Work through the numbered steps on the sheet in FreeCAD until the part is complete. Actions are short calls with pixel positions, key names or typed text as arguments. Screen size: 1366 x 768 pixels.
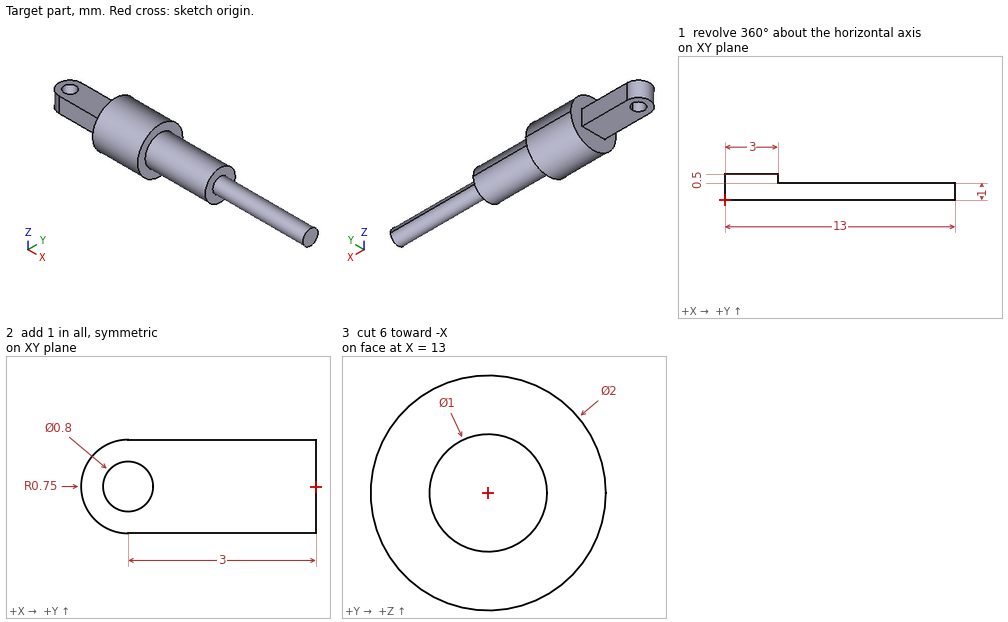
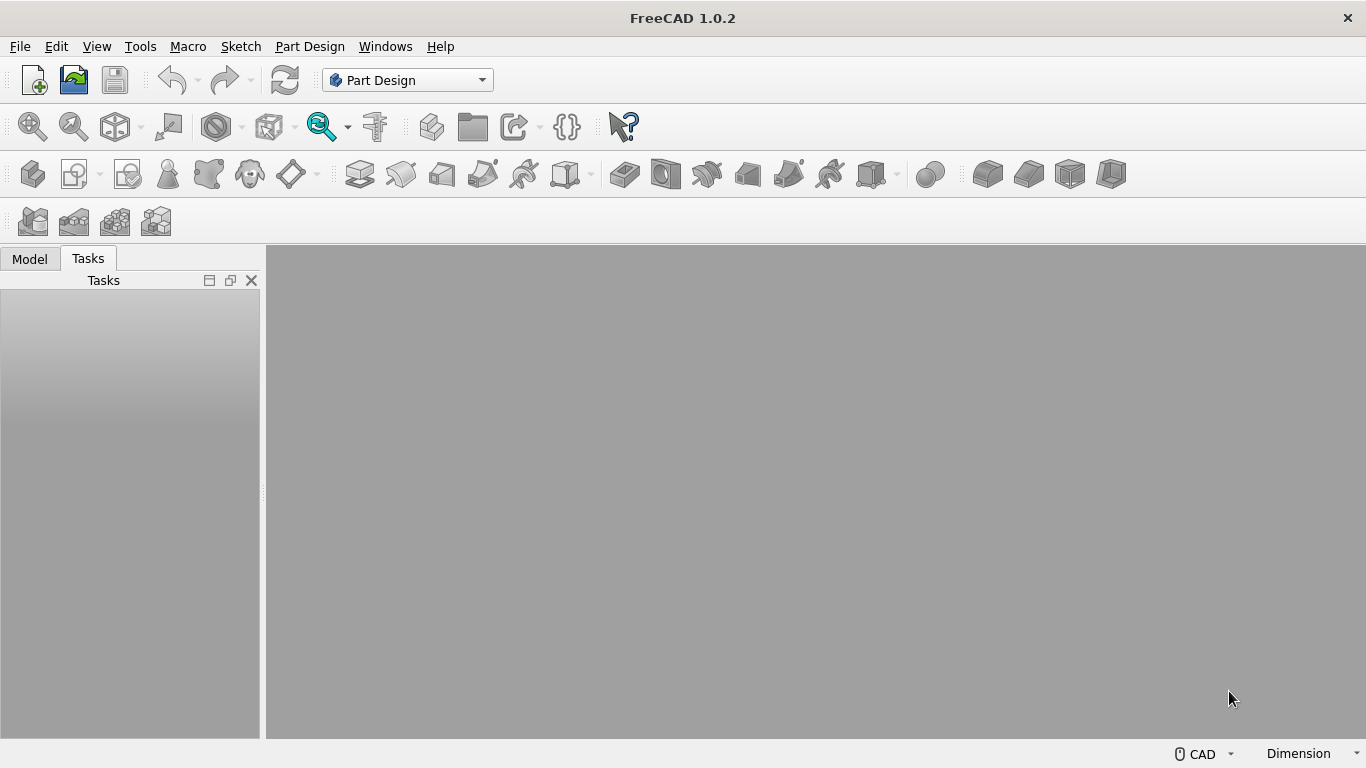
key(ctrl+n)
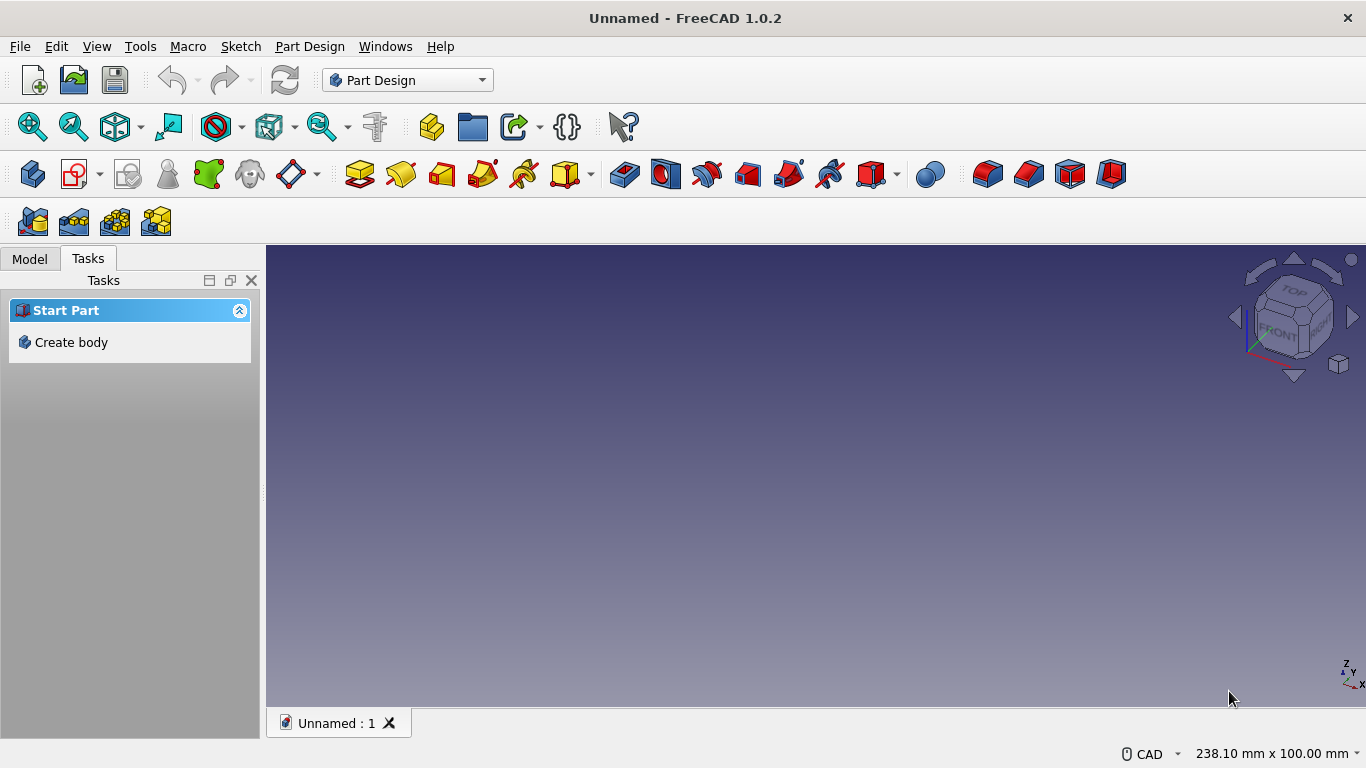
click(74, 174)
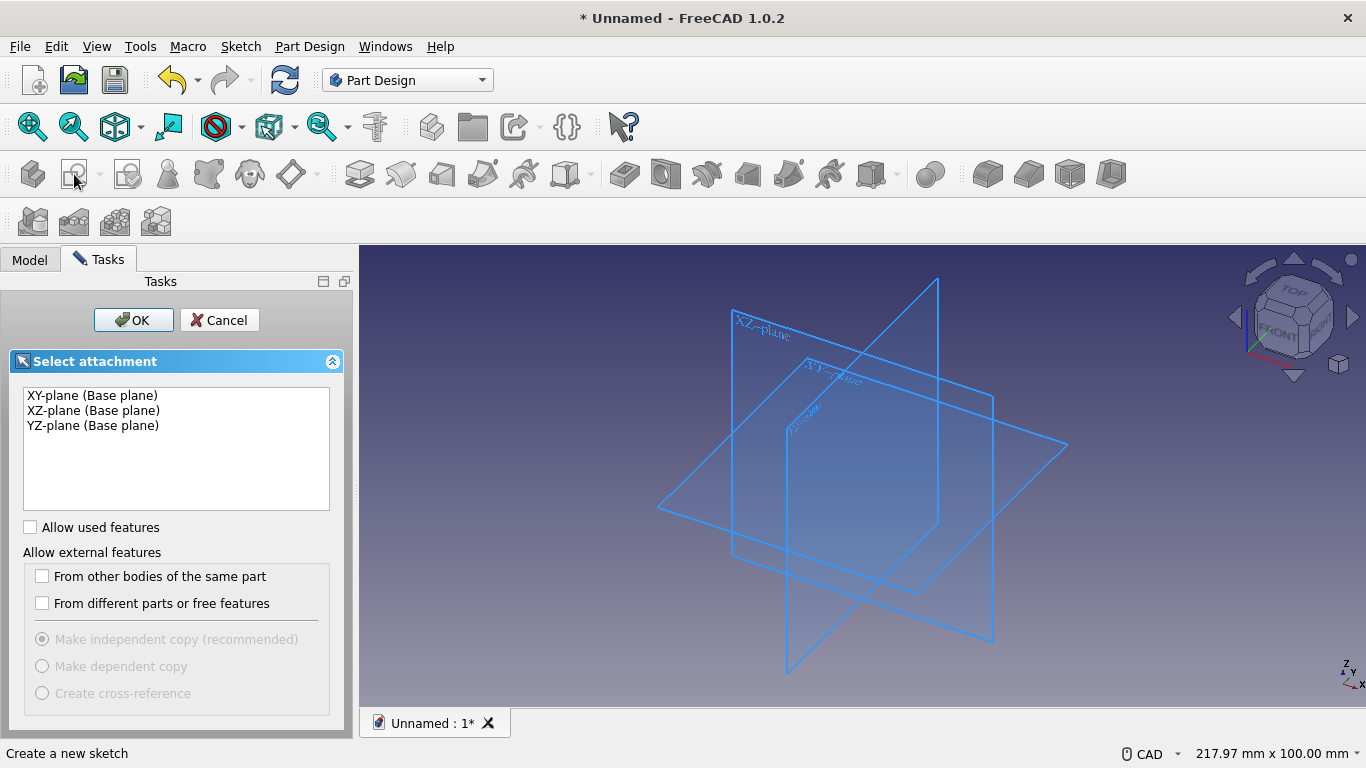
click(84, 396)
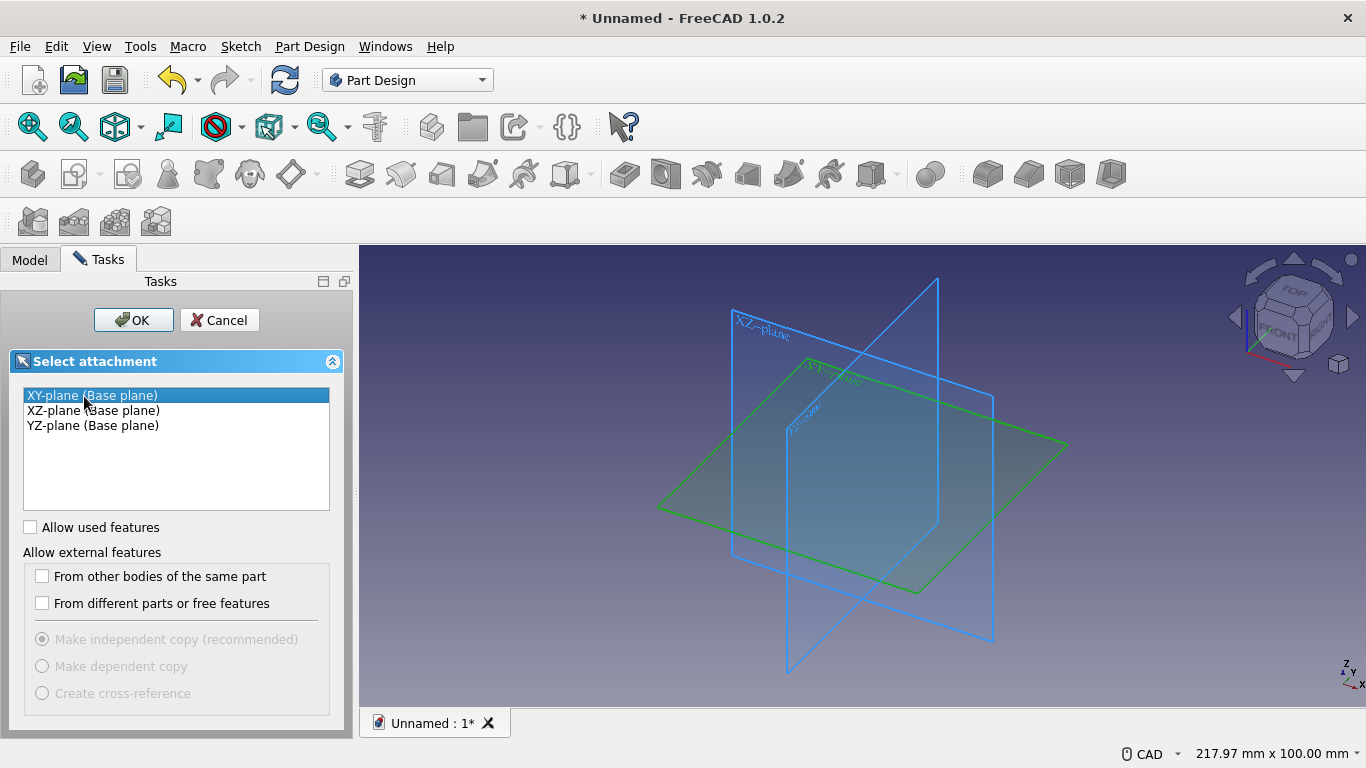
click(134, 320)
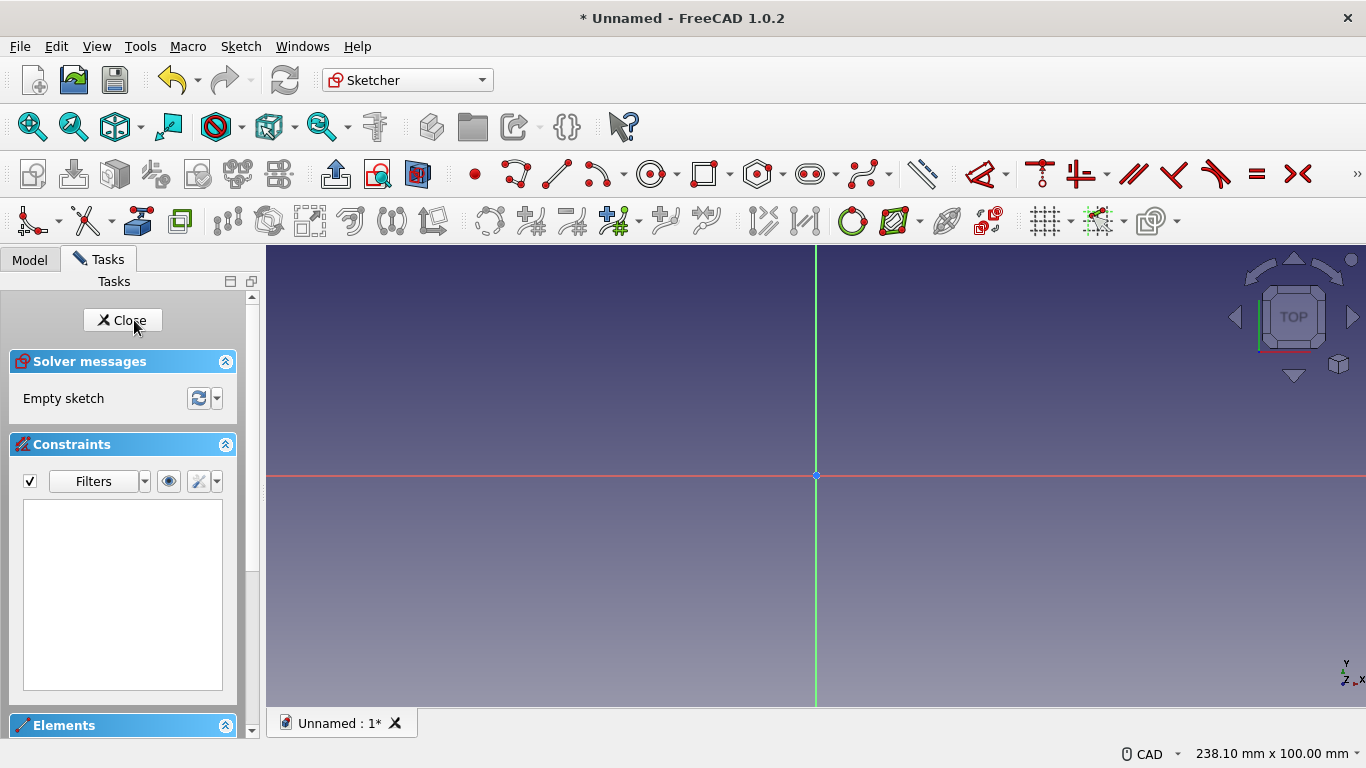
scroll(856, 472, up, 12)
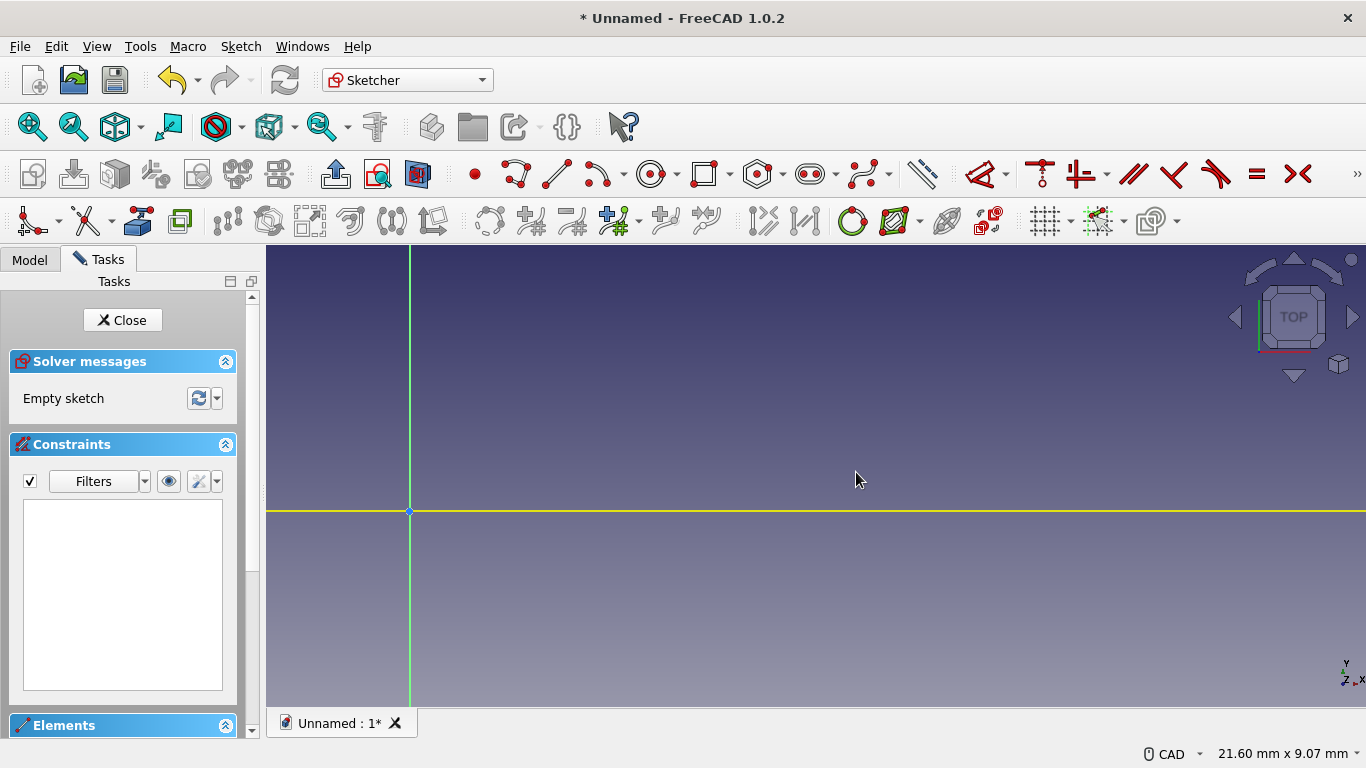
click(516, 174)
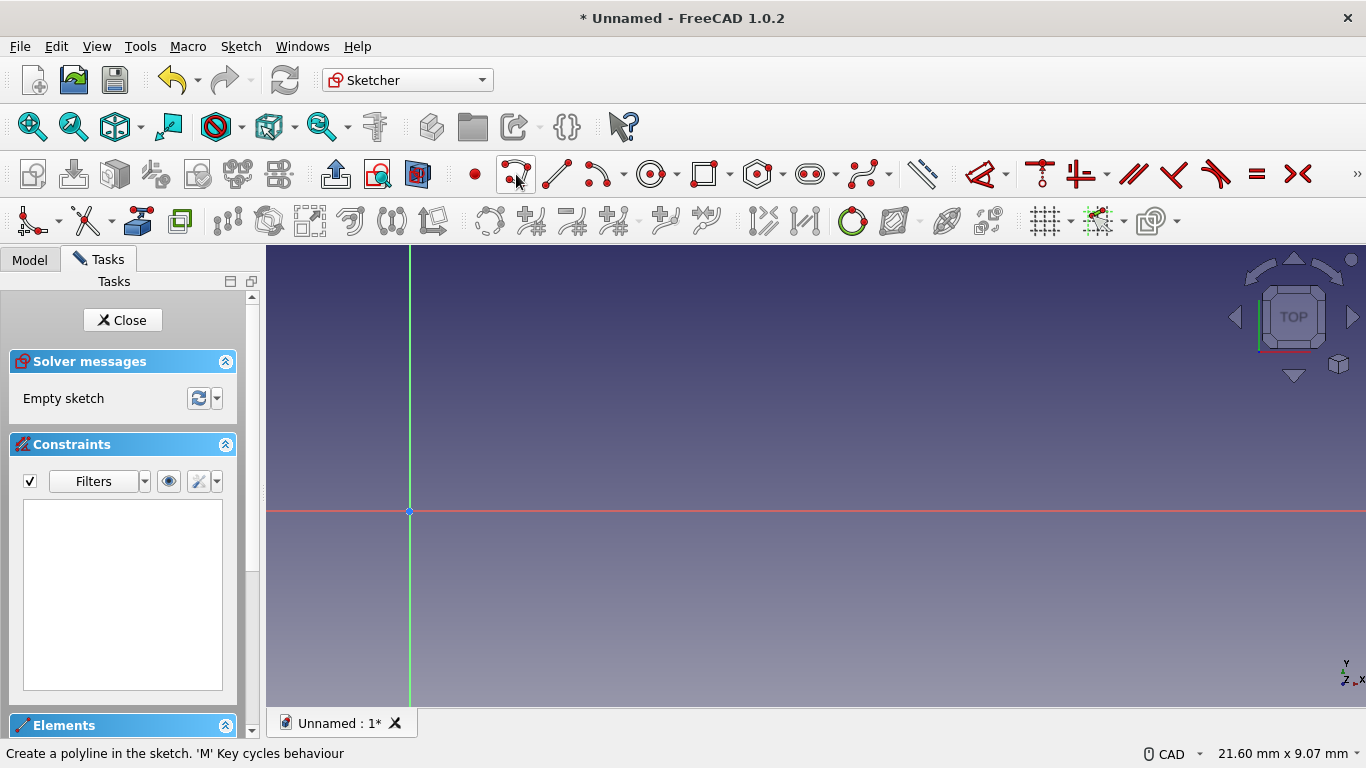
click(410, 511)
click(1072, 502)
click(1072, 460)
click(562, 460)
click(562, 435)
click(419, 435)
click(410, 511)
key(Escape)
key(Escape)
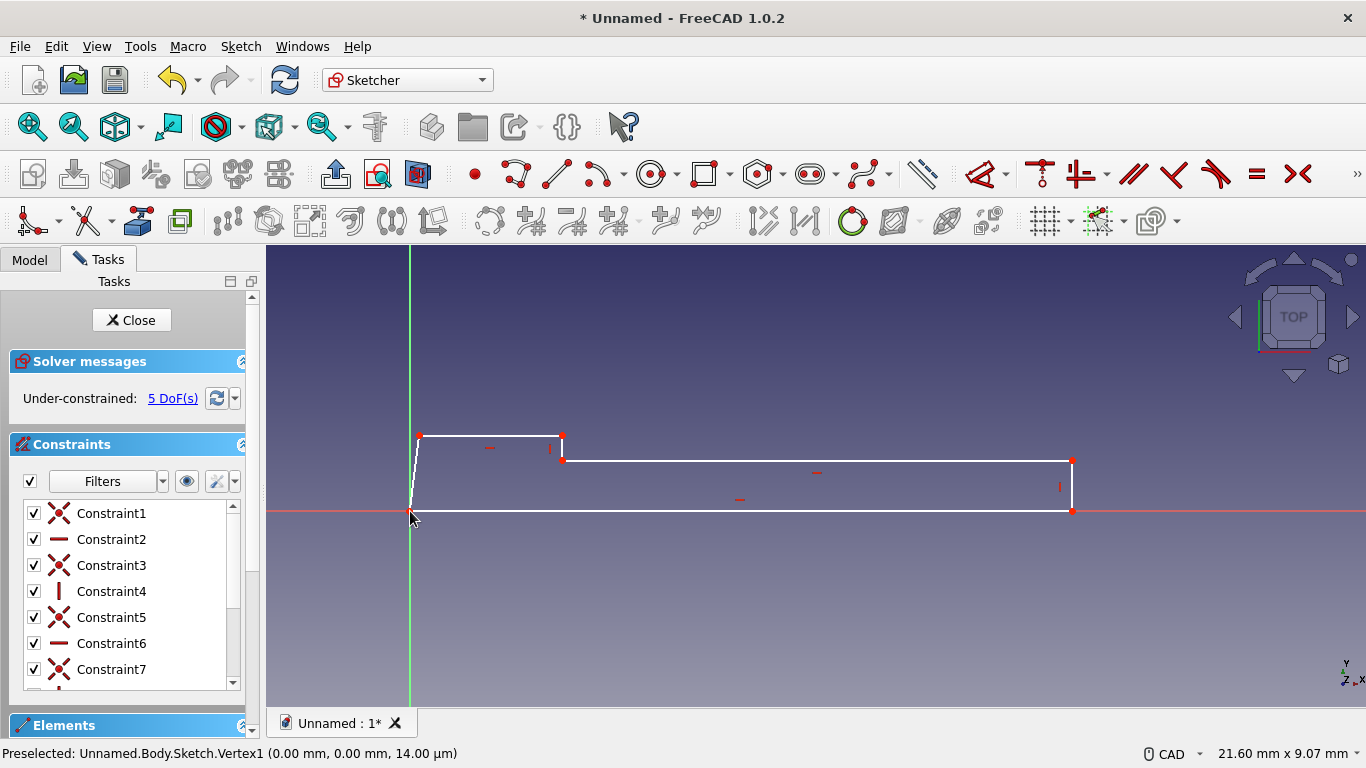
click(412, 489)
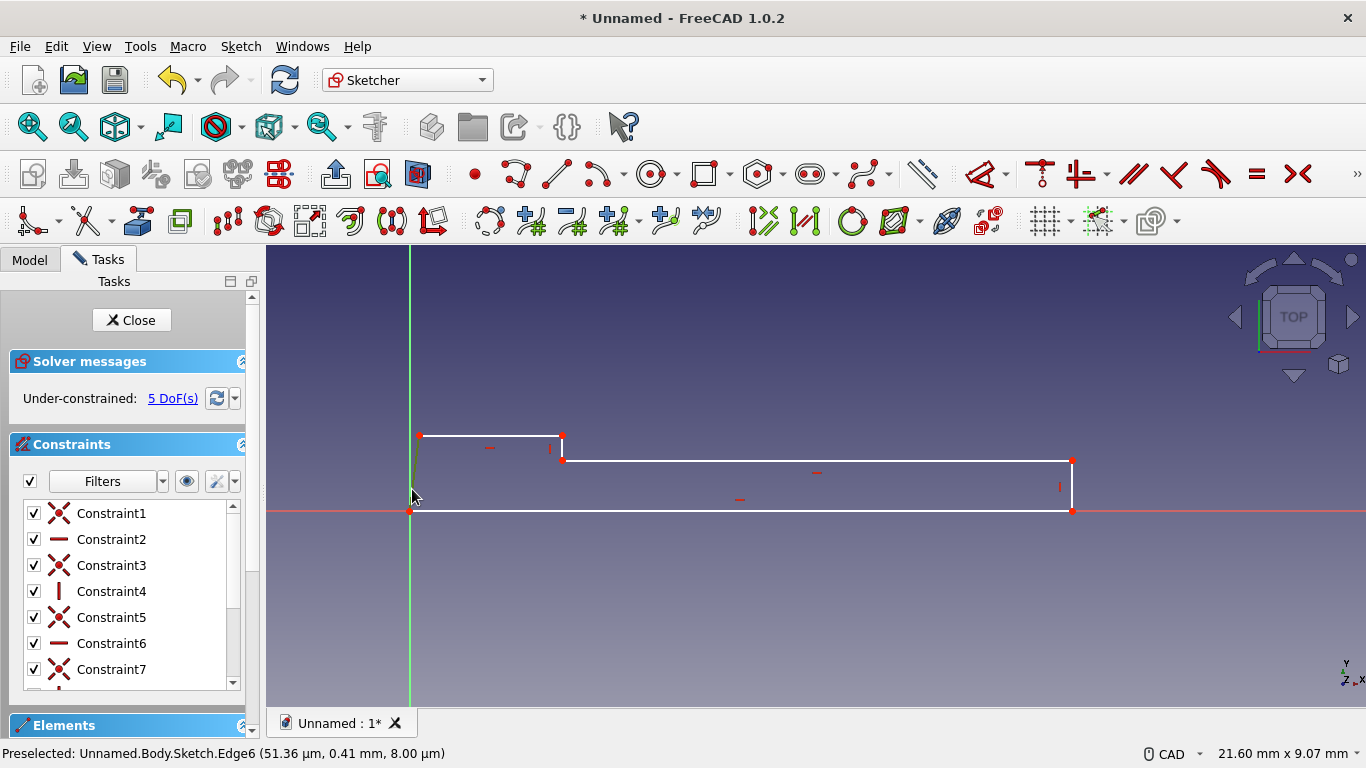
key(v)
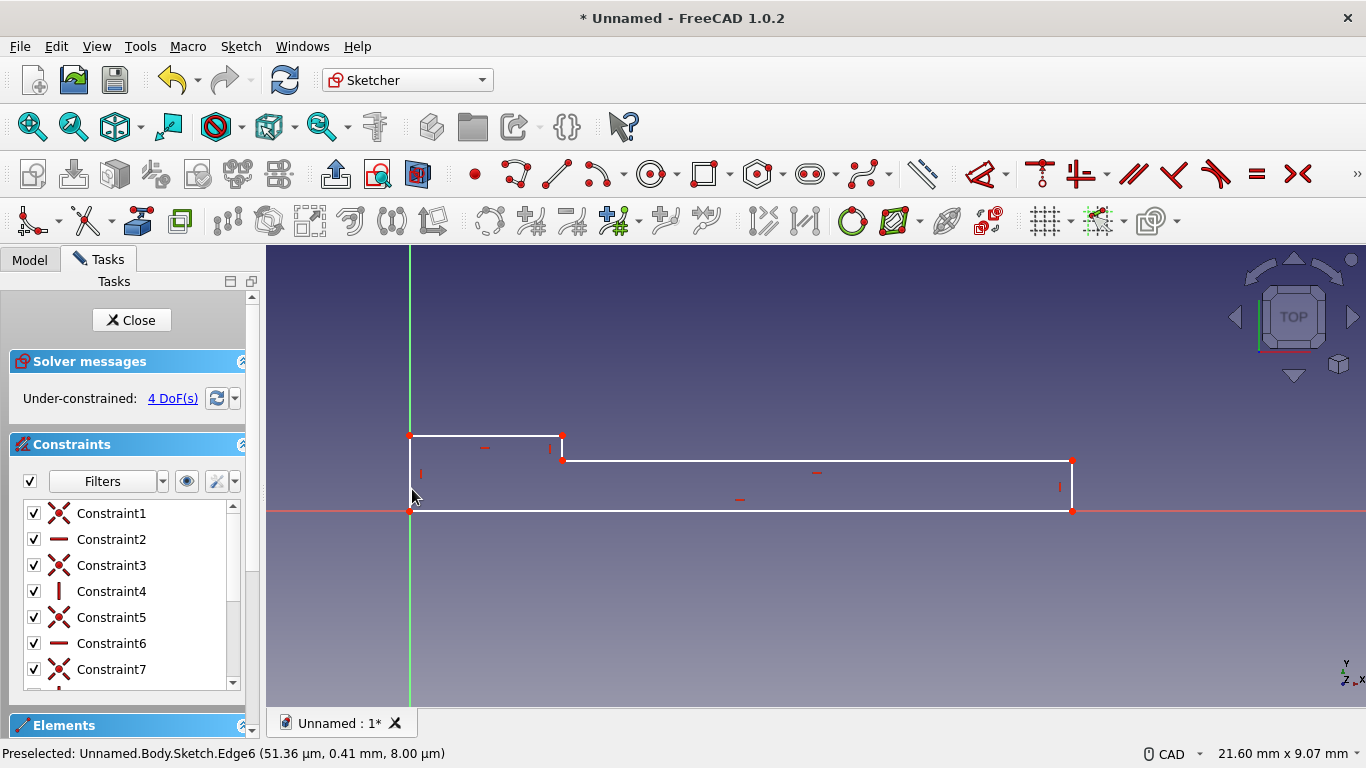
key(d)